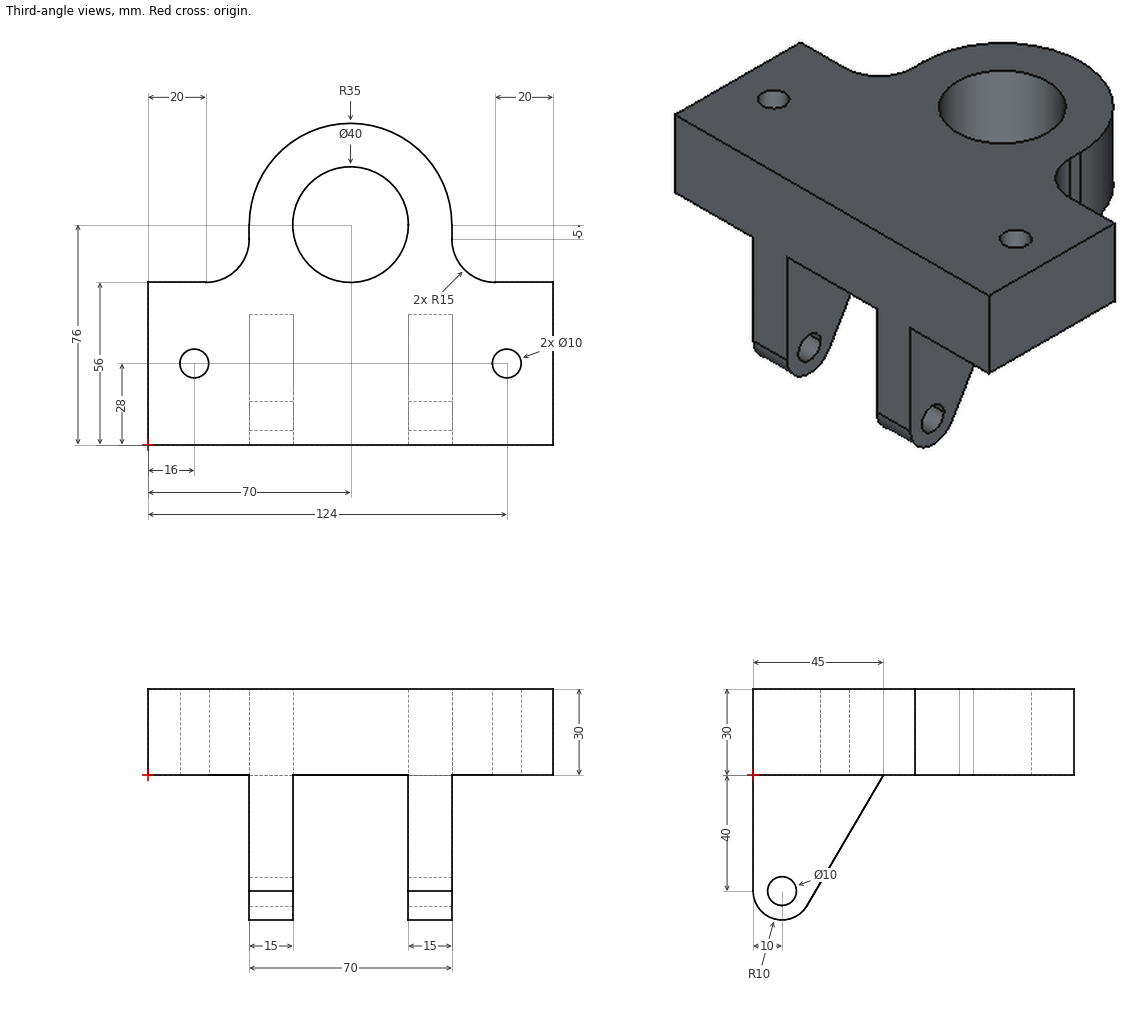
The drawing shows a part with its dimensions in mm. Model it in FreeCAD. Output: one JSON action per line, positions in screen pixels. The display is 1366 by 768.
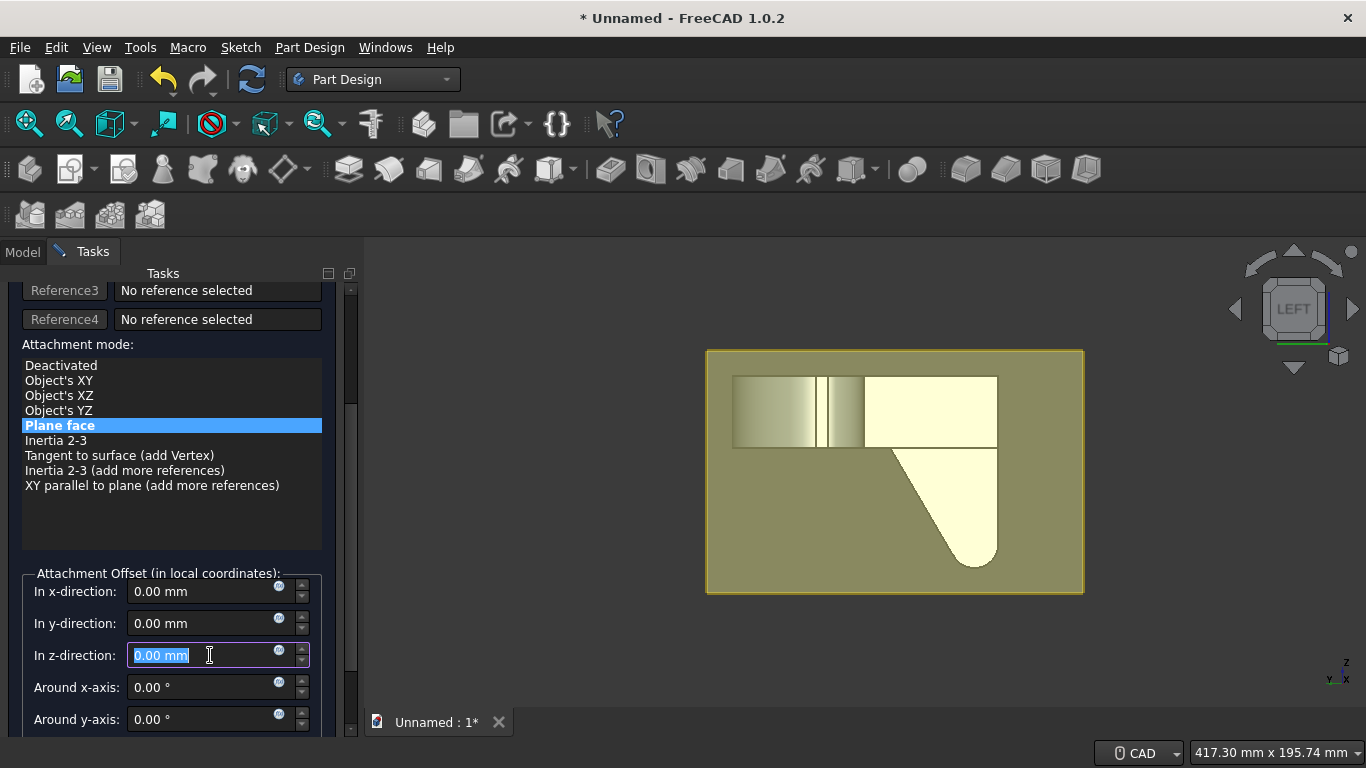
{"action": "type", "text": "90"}
{"action": "key", "text": "Tab"}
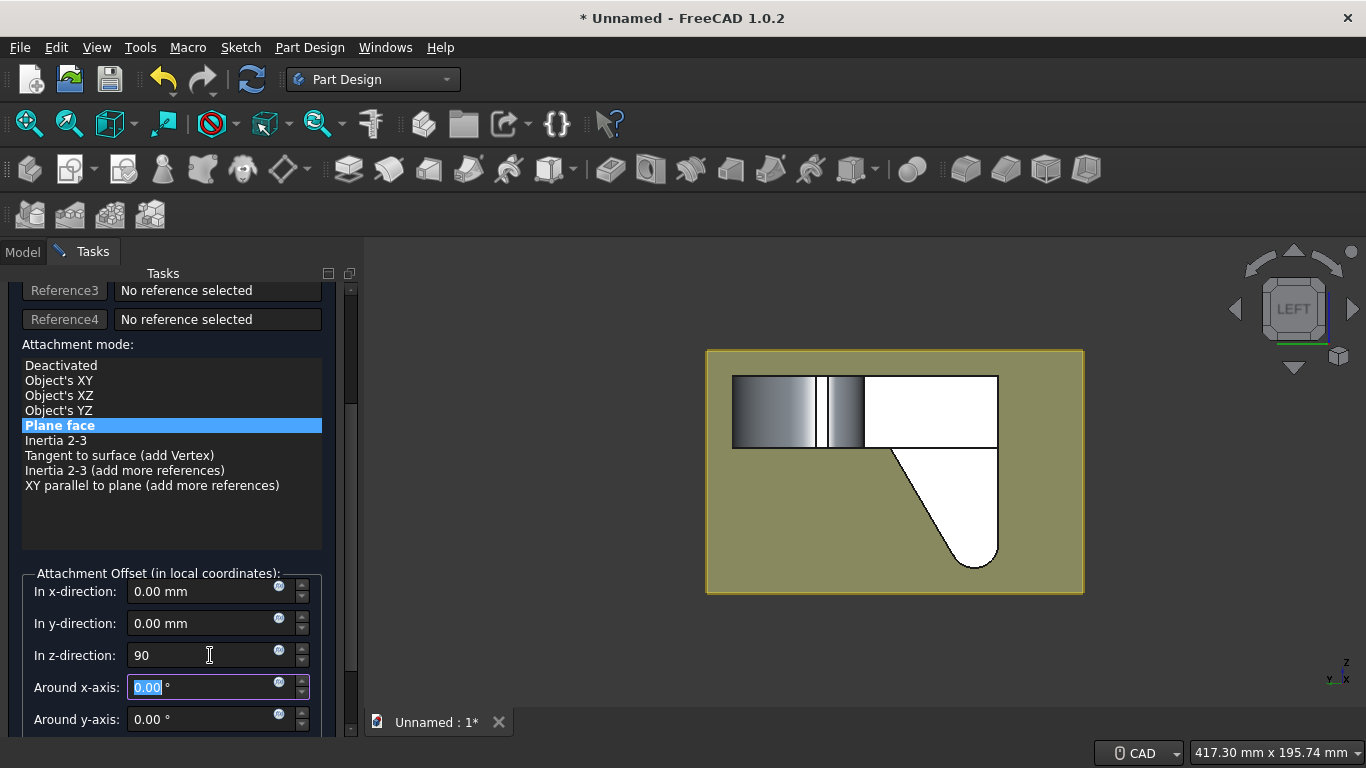
{"action": "scroll", "coordinate": [351, 510], "scroll_direction": "up", "scroll_amount": 4}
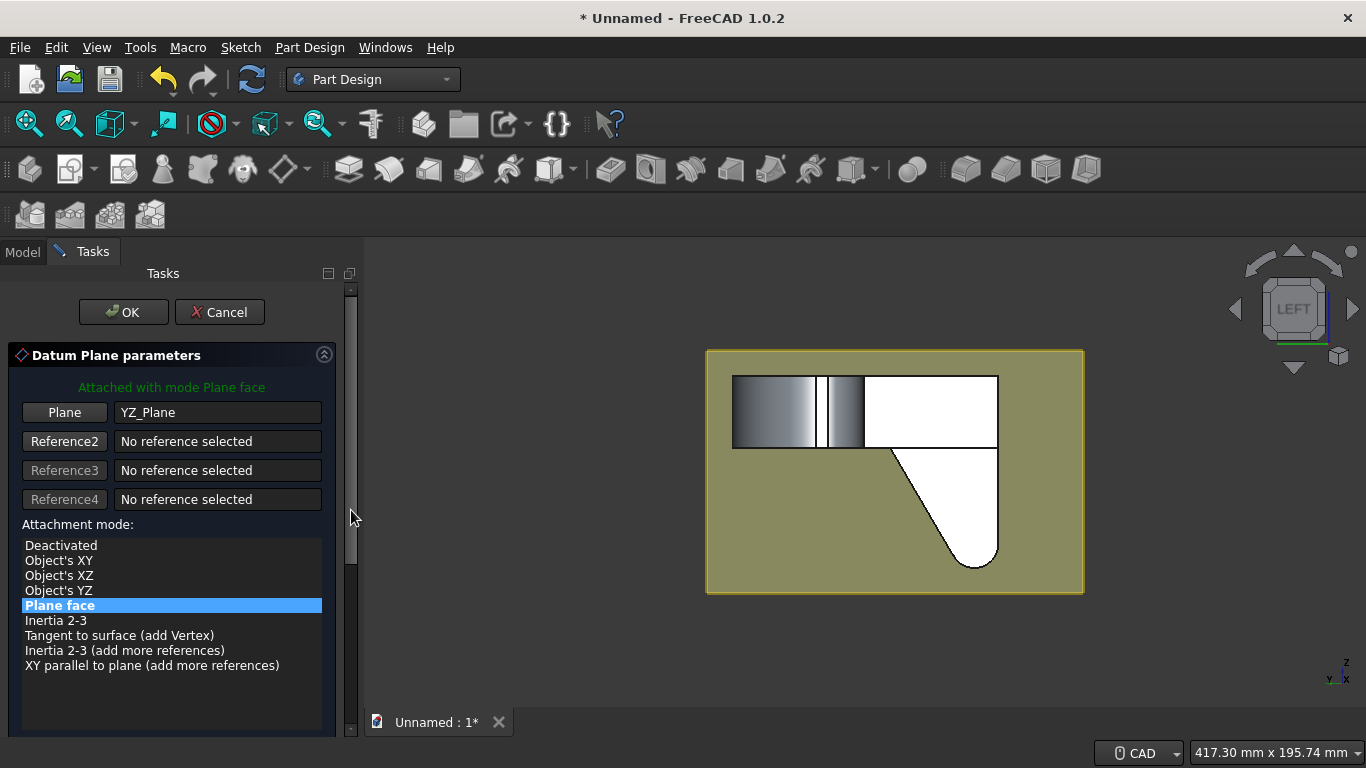
{"action": "left_click", "coordinate": [124, 312]}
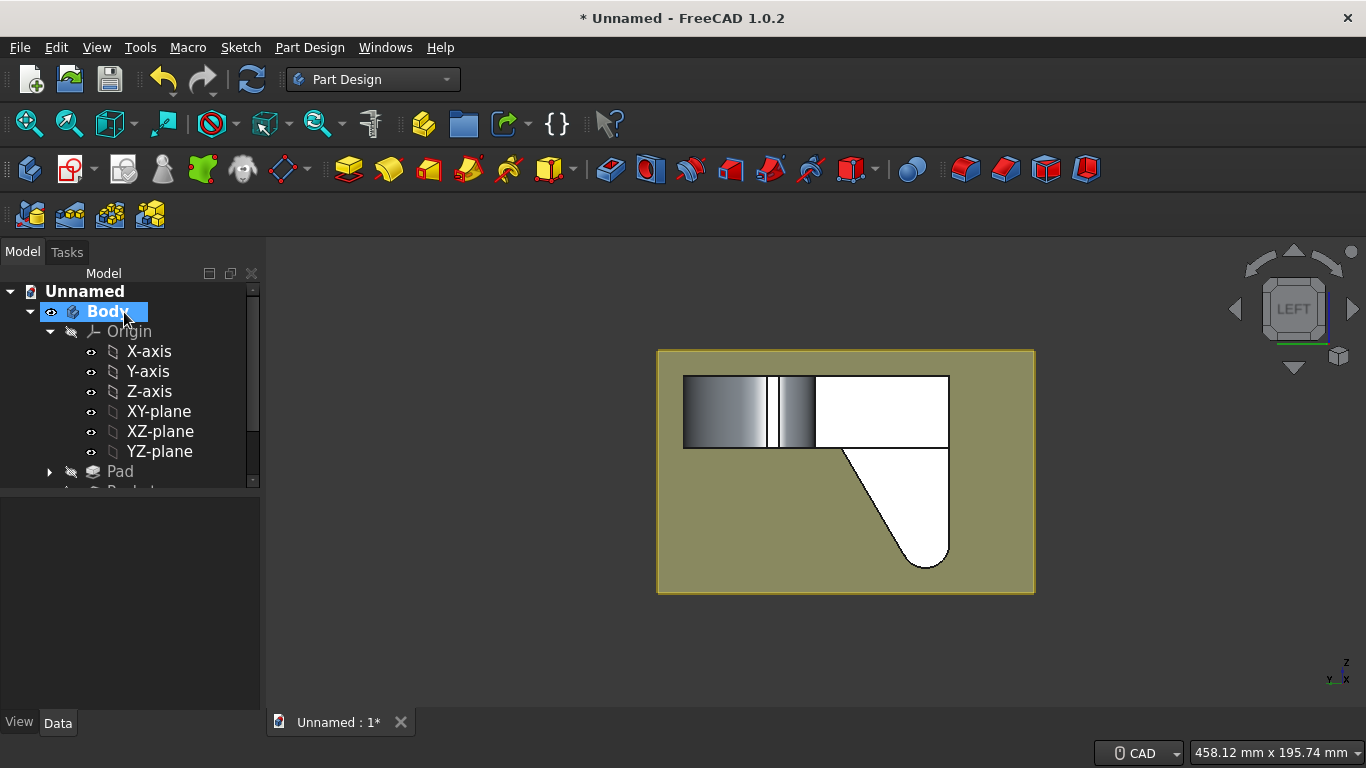
{"action": "scroll", "coordinate": [100, 387], "scroll_direction": "down", "scroll_amount": 3}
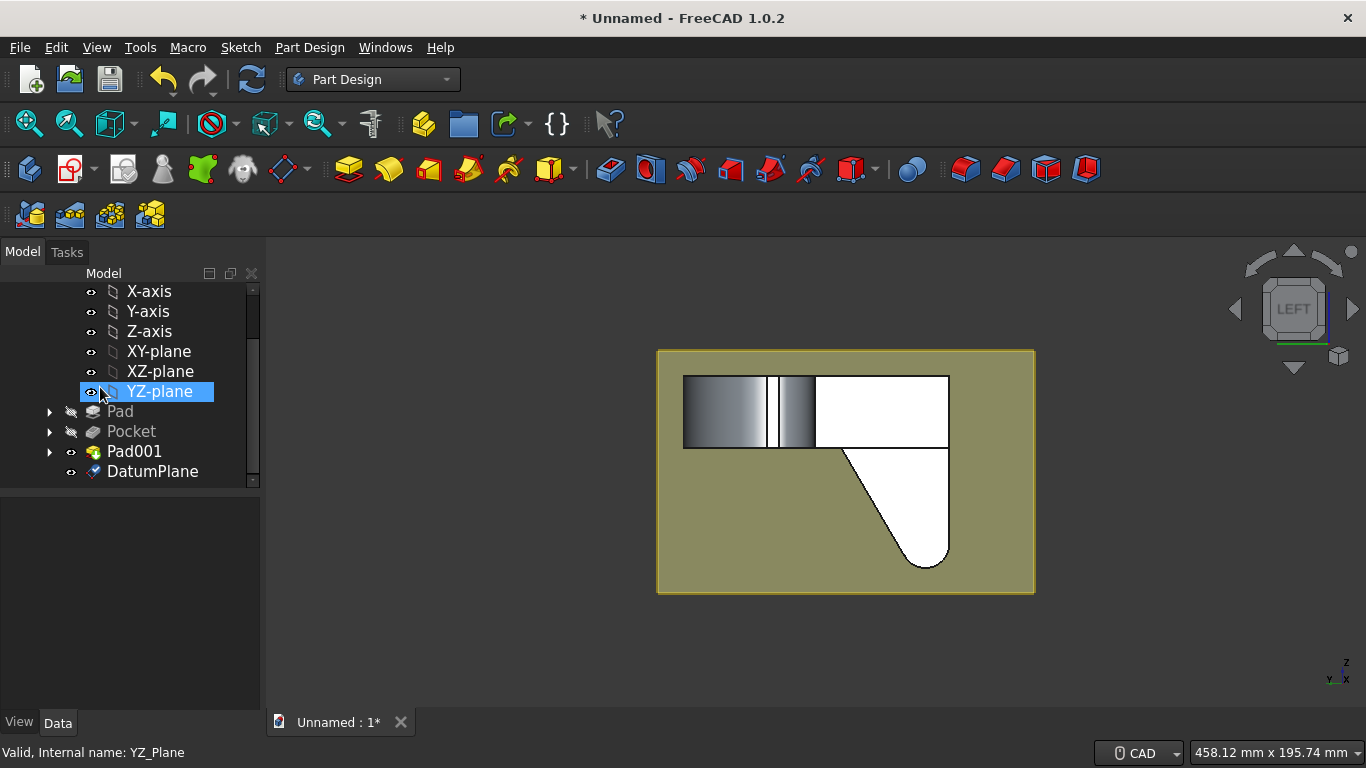
{"action": "left_click", "coordinate": [116, 472]}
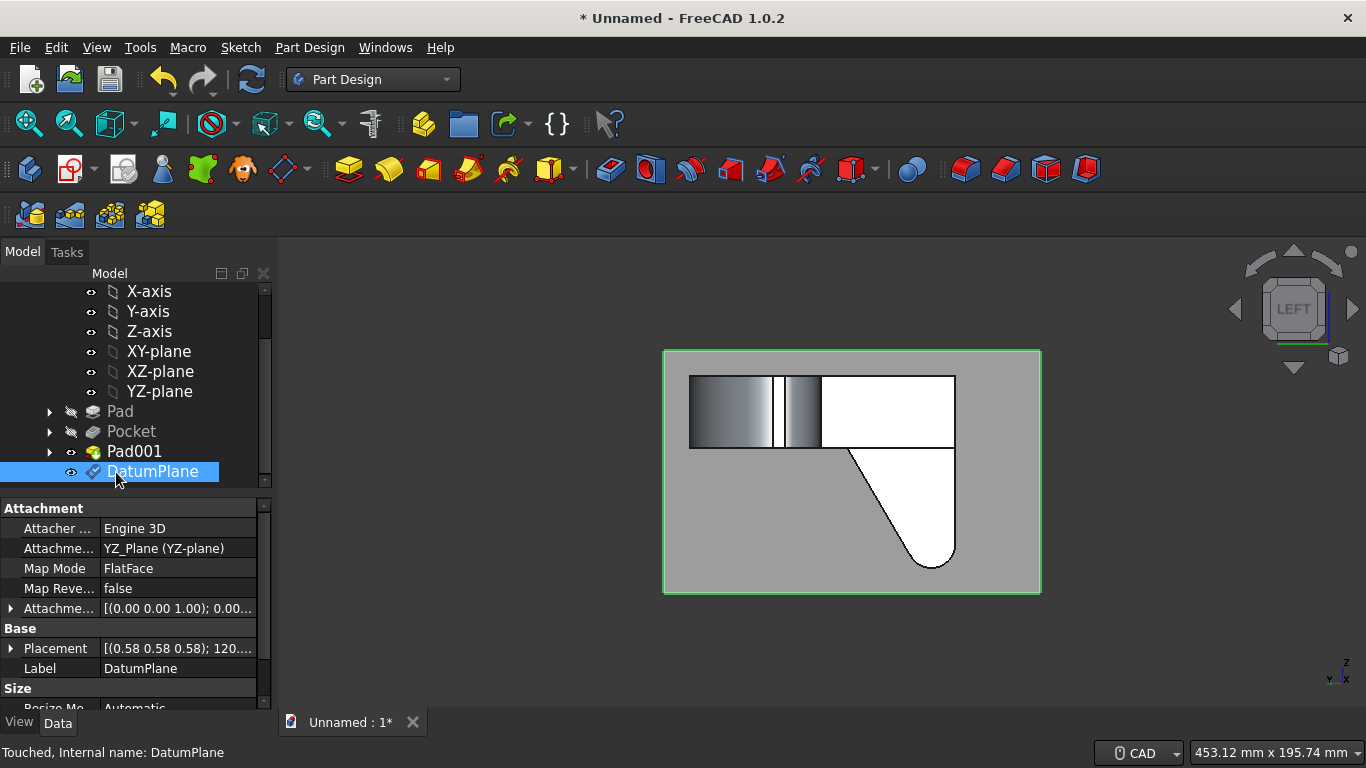
{"action": "left_click", "coordinate": [70, 170]}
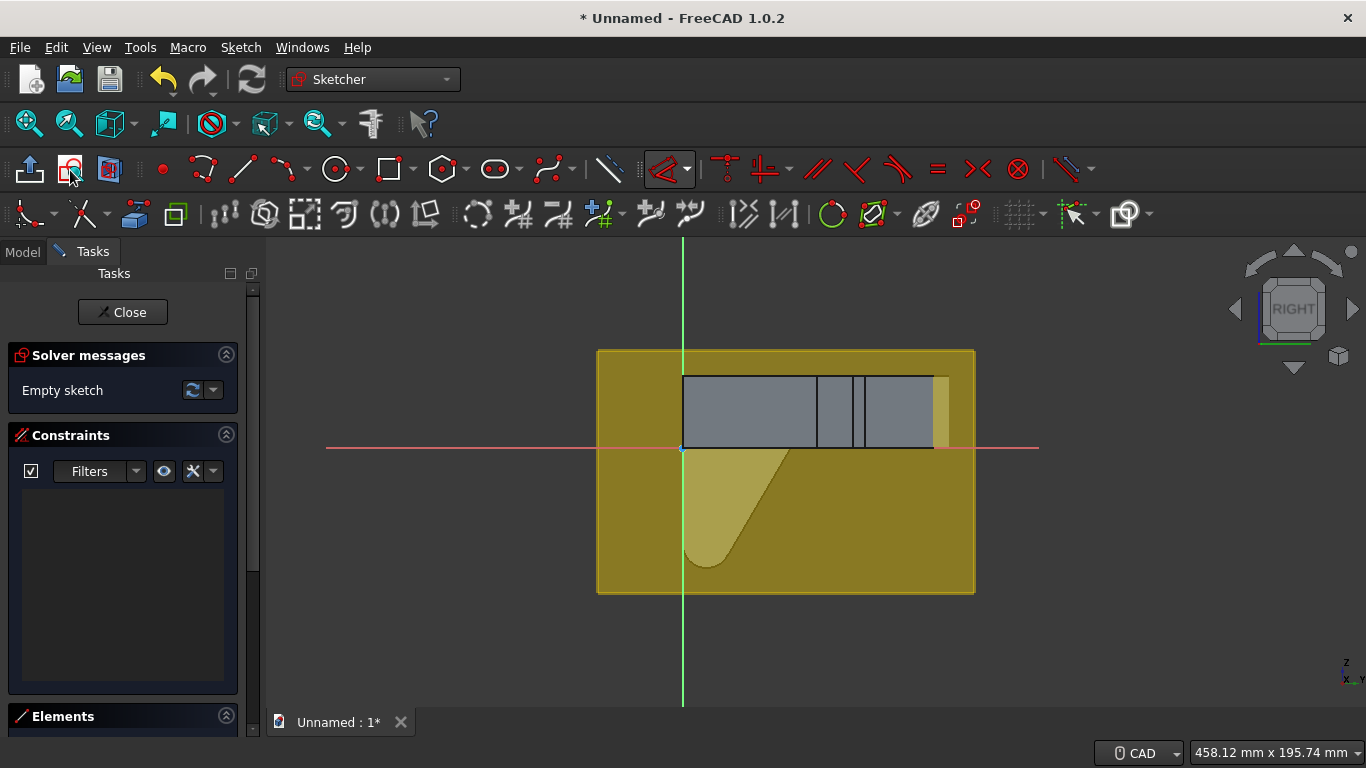
{"action": "left_click", "coordinate": [110, 170]}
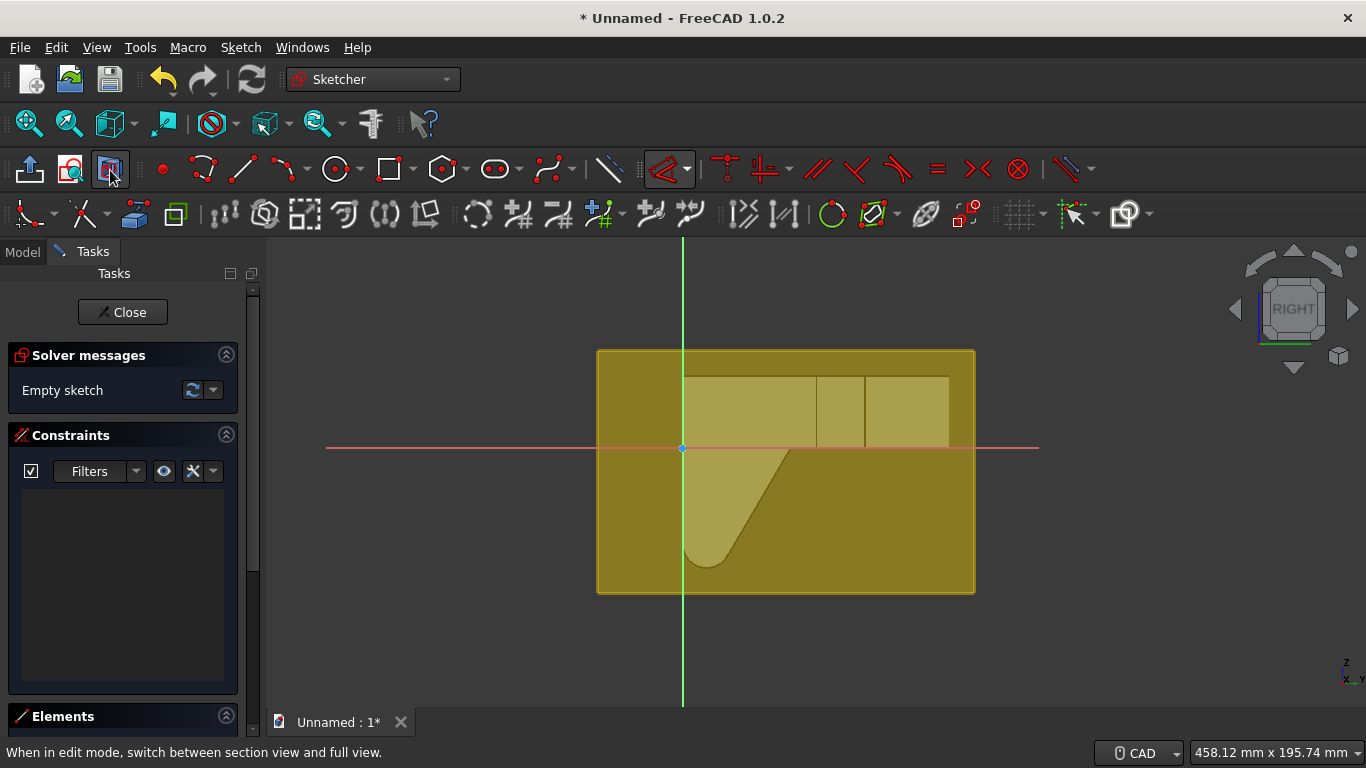
{"action": "scroll", "coordinate": [728, 537], "scroll_direction": "up", "scroll_amount": 4}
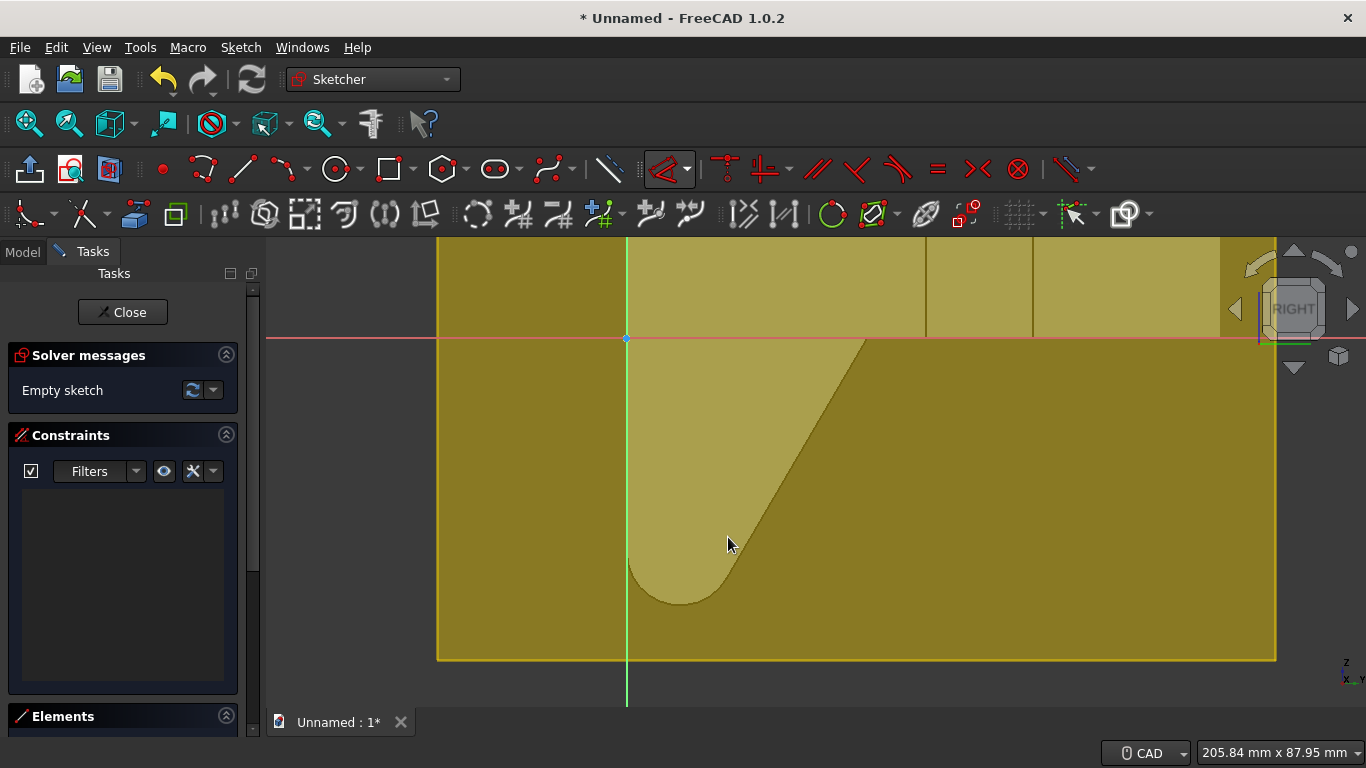
{"action": "key", "text": "g m"}